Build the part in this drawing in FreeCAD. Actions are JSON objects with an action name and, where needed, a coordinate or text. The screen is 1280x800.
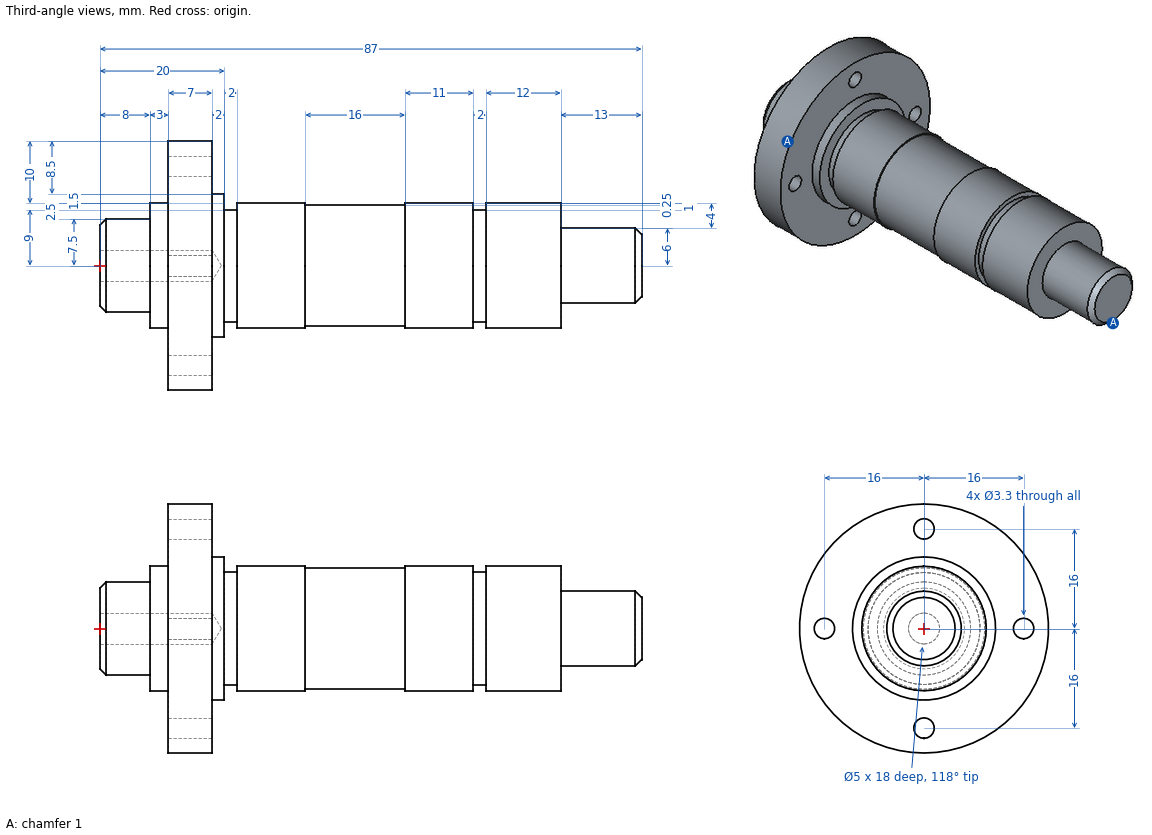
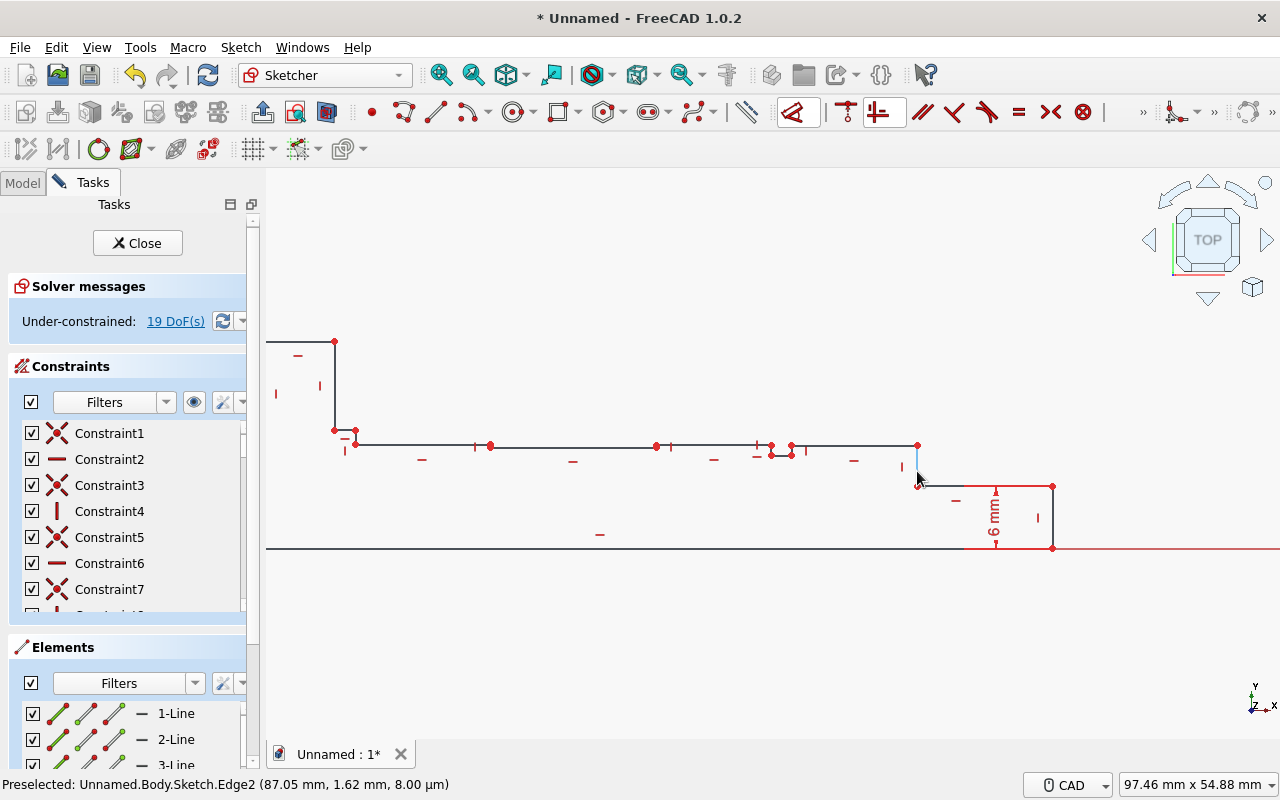
{"action": "left_click", "coordinate": [917, 470]}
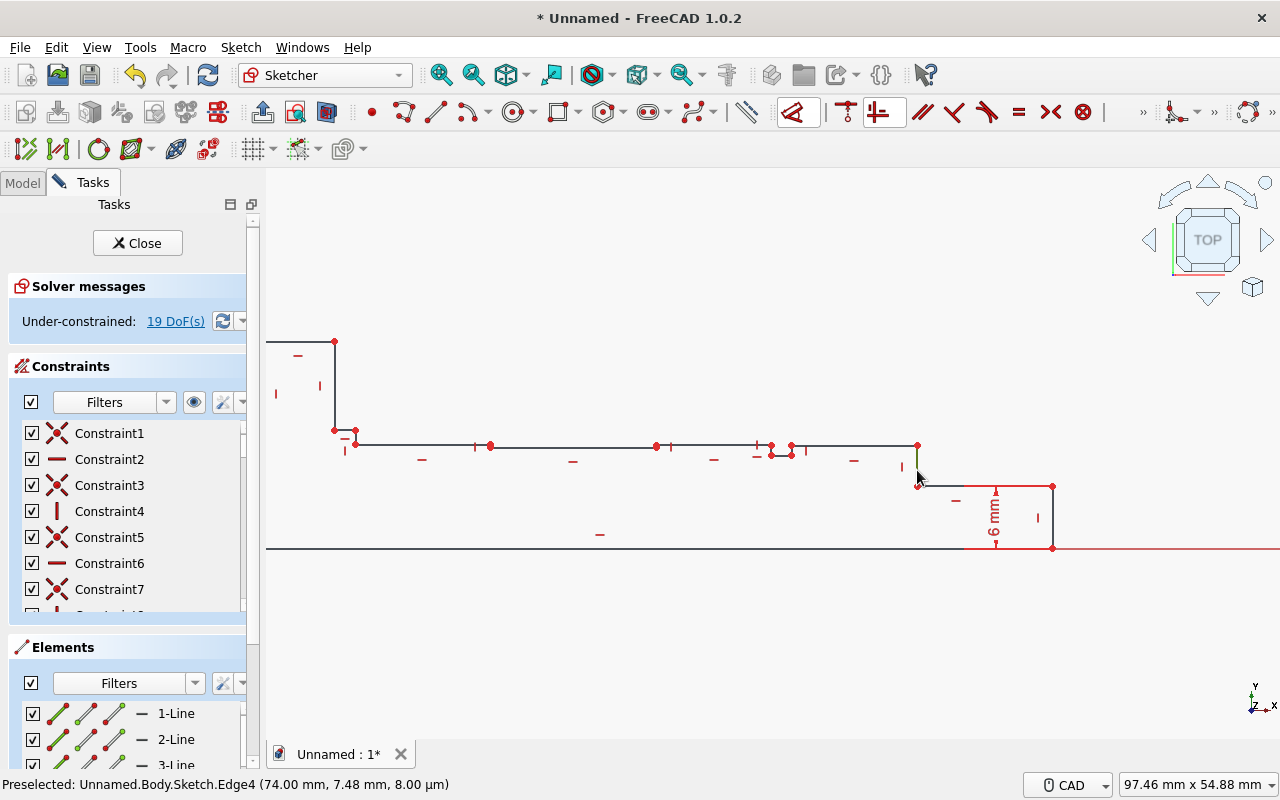
{"action": "key", "text": "i"}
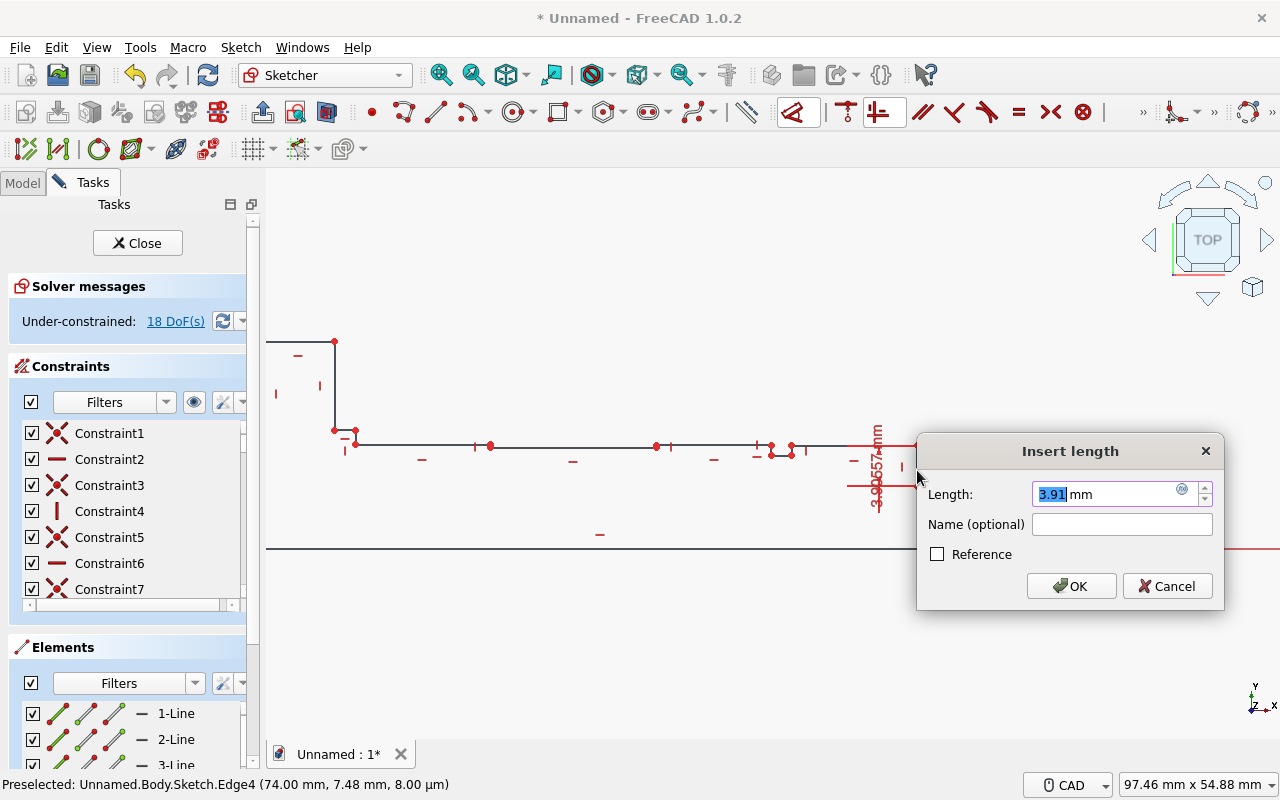
{"action": "type", "text": "4"}
{"action": "key", "text": "Return"}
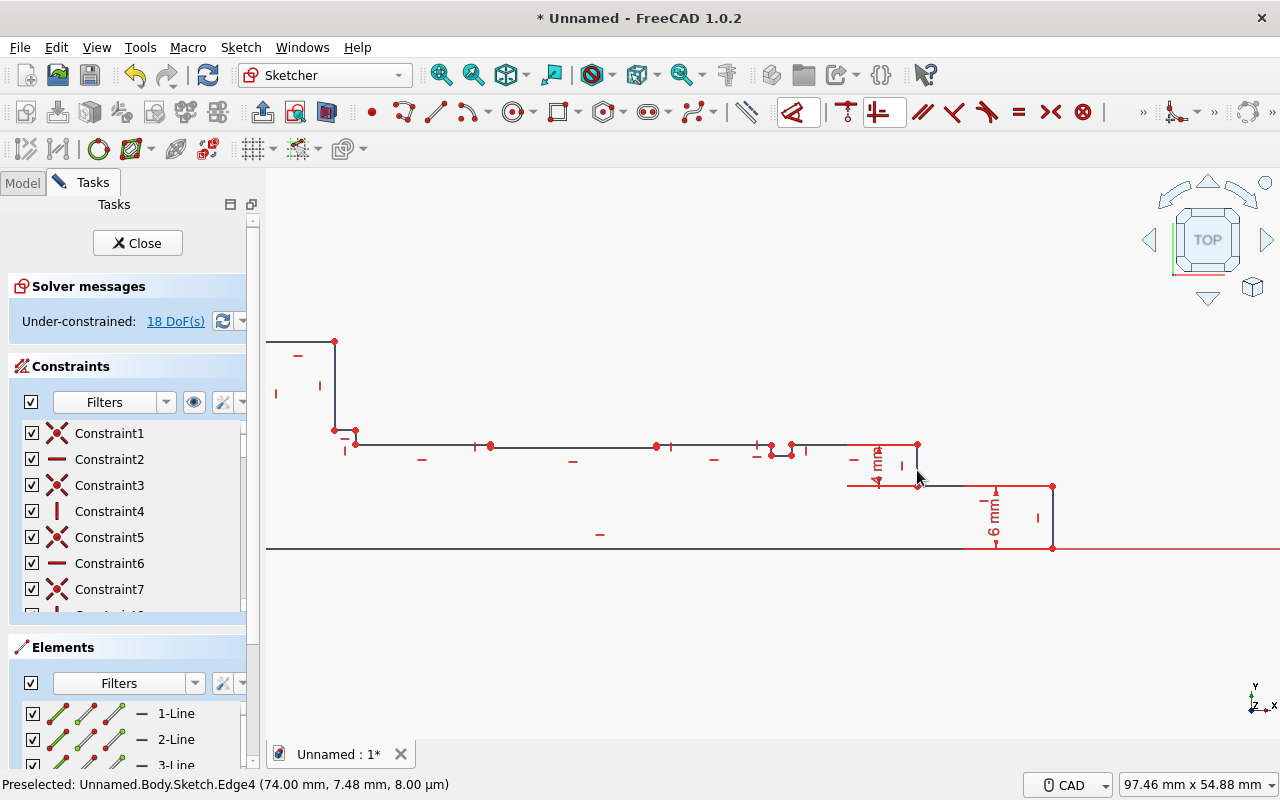
{"action": "scroll", "coordinate": [792, 450], "scroll_direction": "up", "scroll_amount": 7}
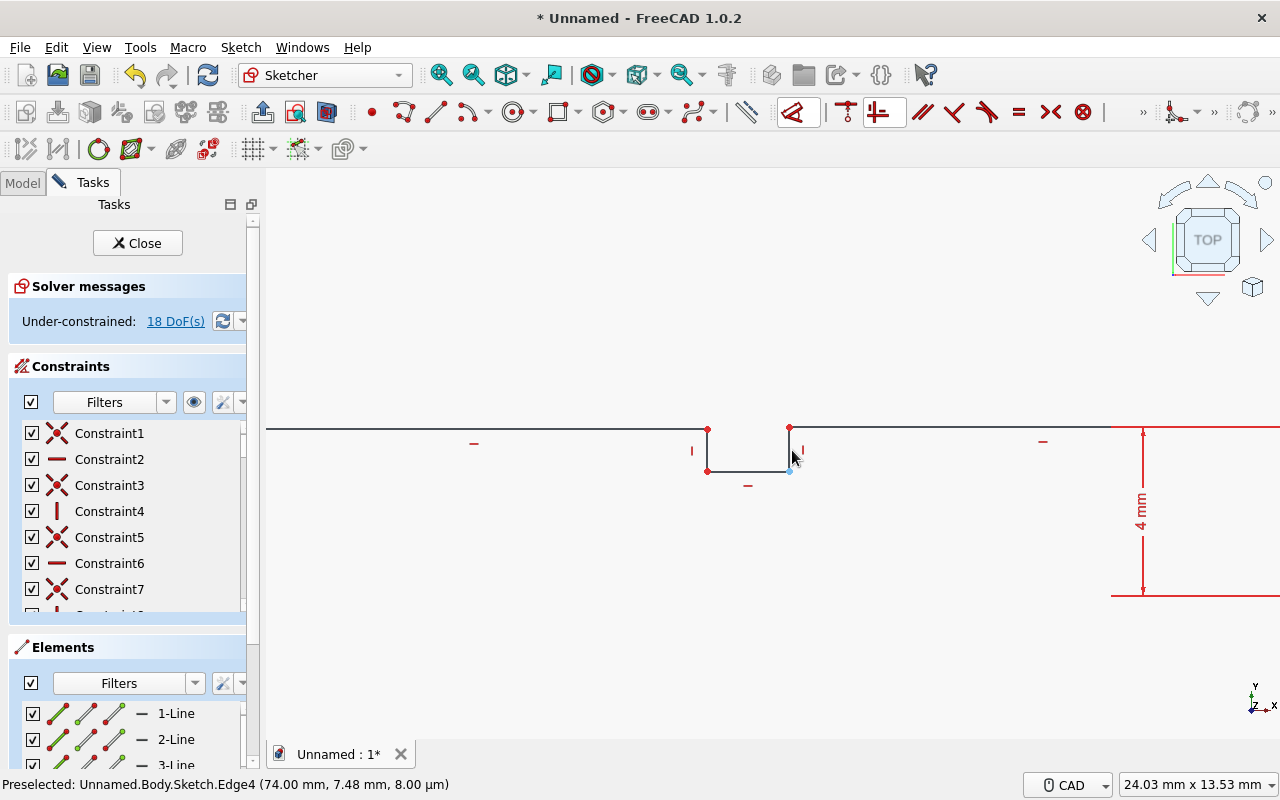
{"action": "left_click", "coordinate": [789, 449]}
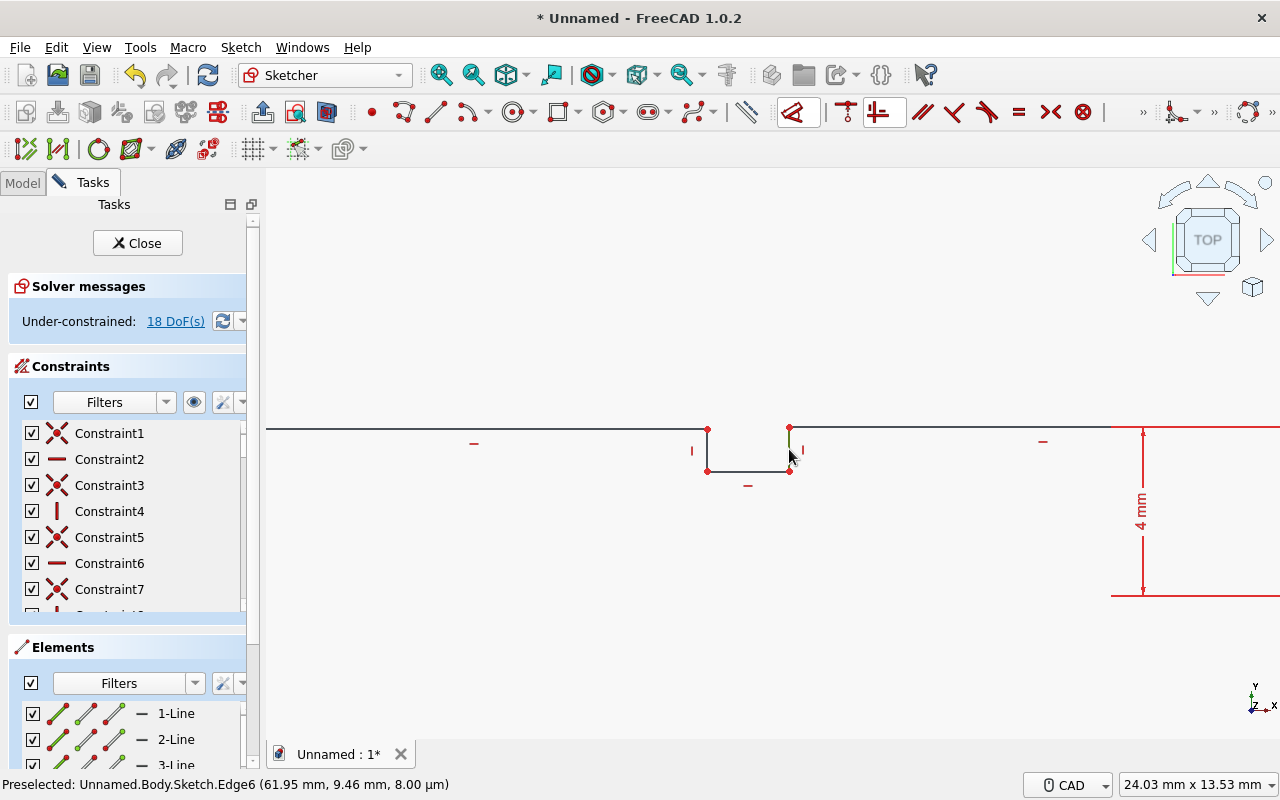
{"action": "key", "text": "i"}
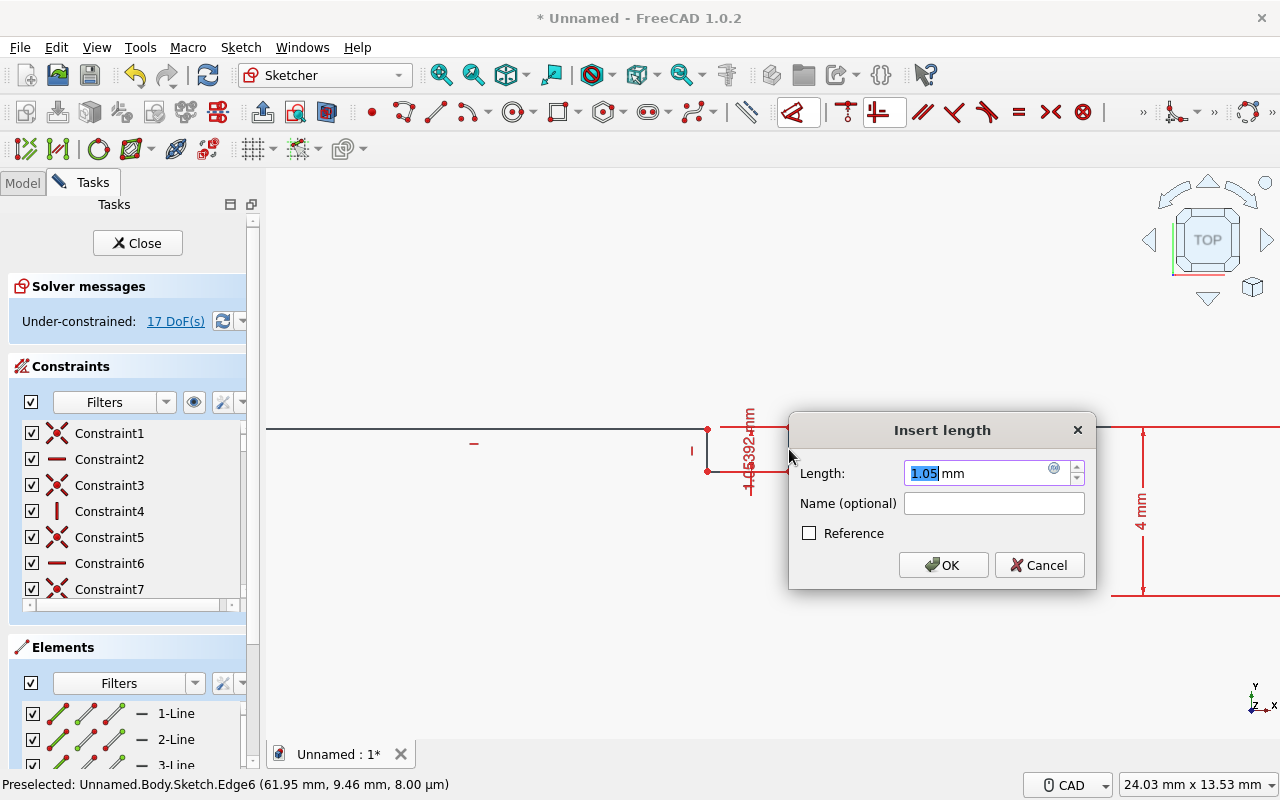
{"action": "type", "text": "1"}
{"action": "key", "text": "Return"}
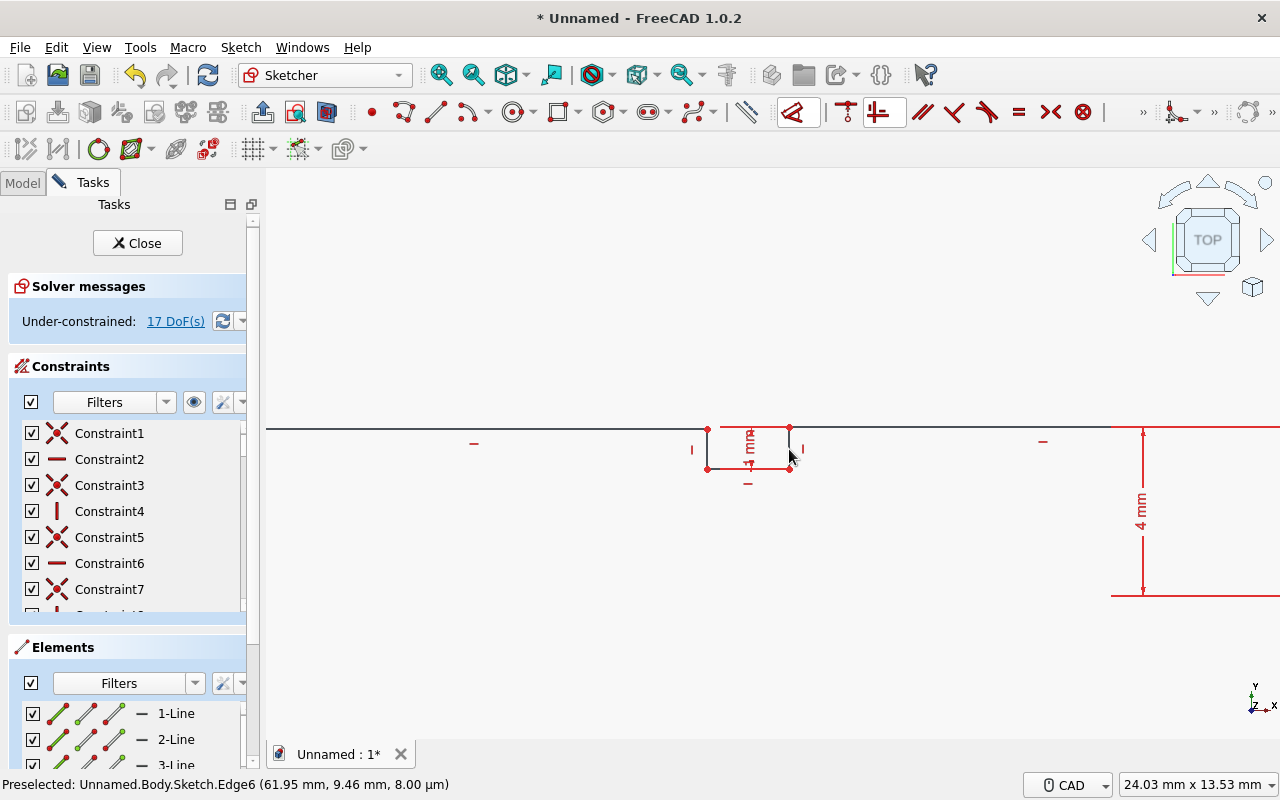
{"action": "left_click", "coordinate": [765, 469]}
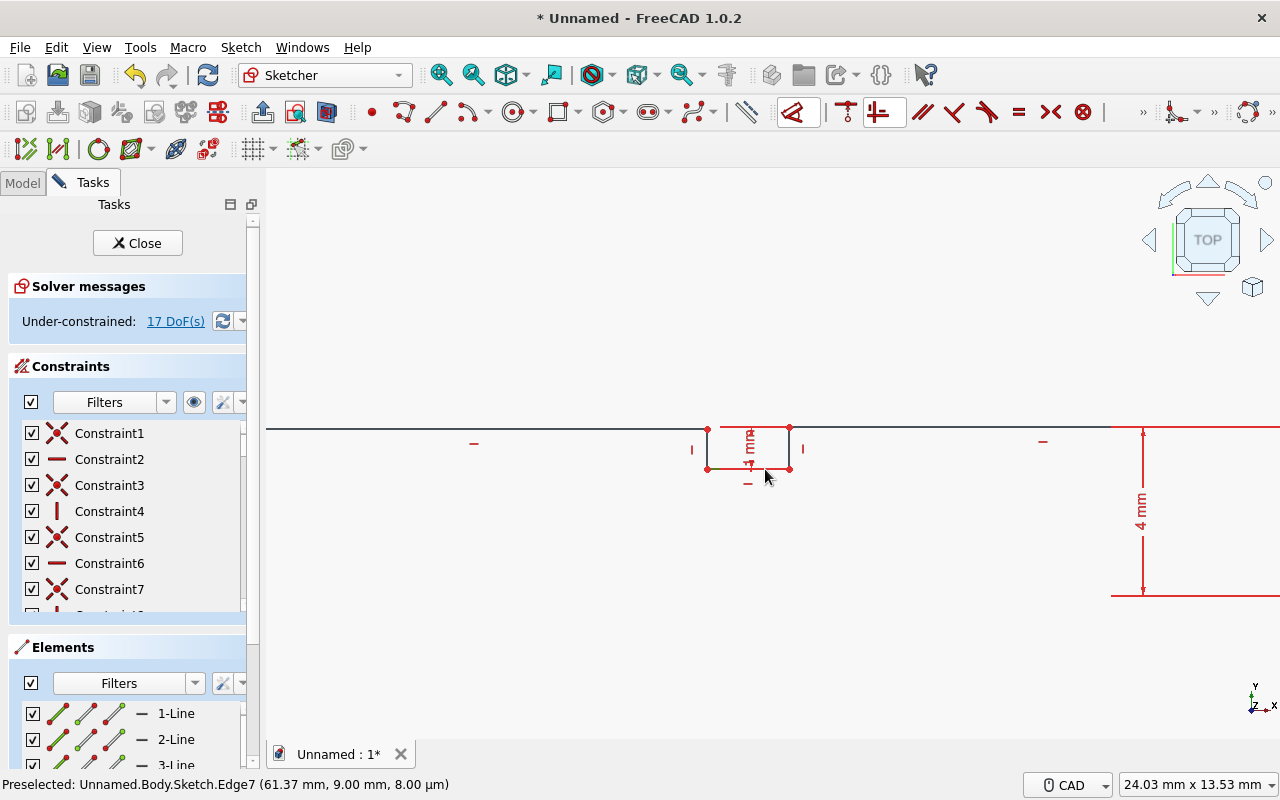
{"action": "key", "text": "l"}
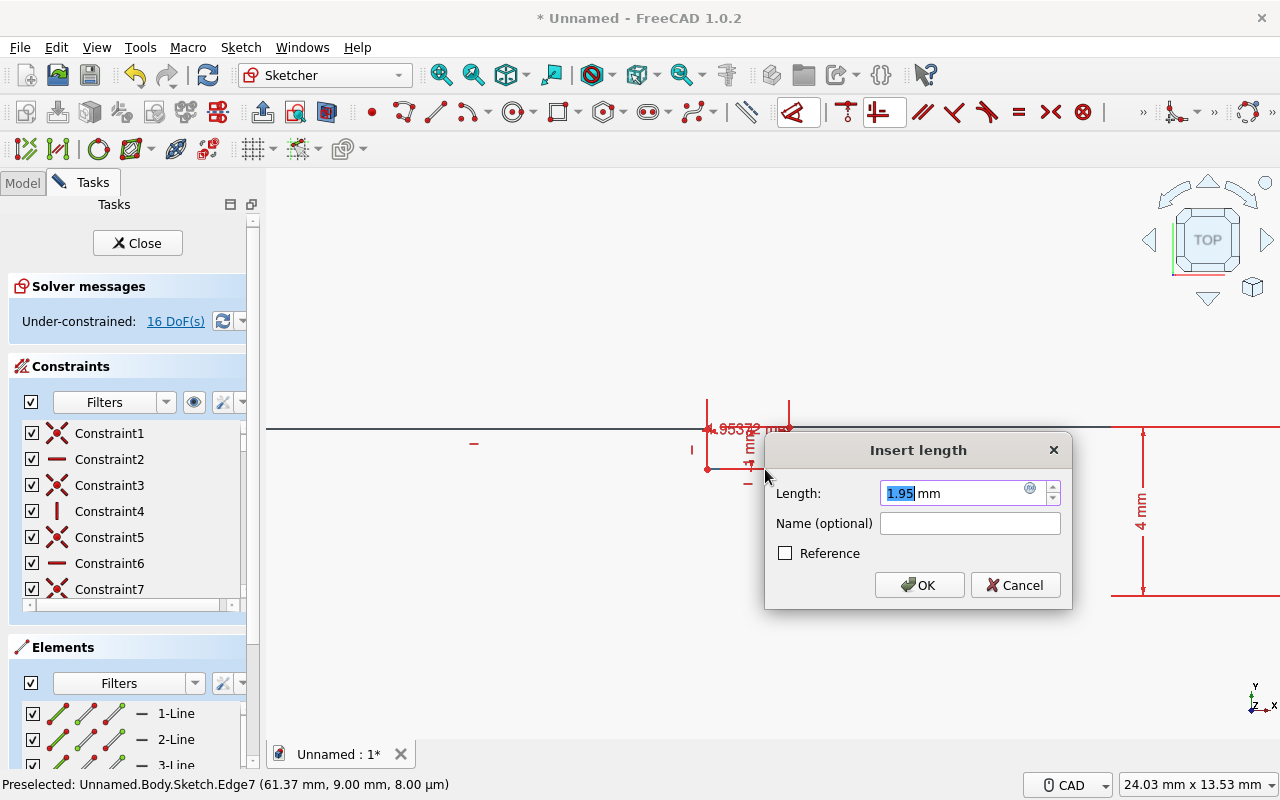
{"action": "type", "text": "2"}
{"action": "key", "text": "Return"}